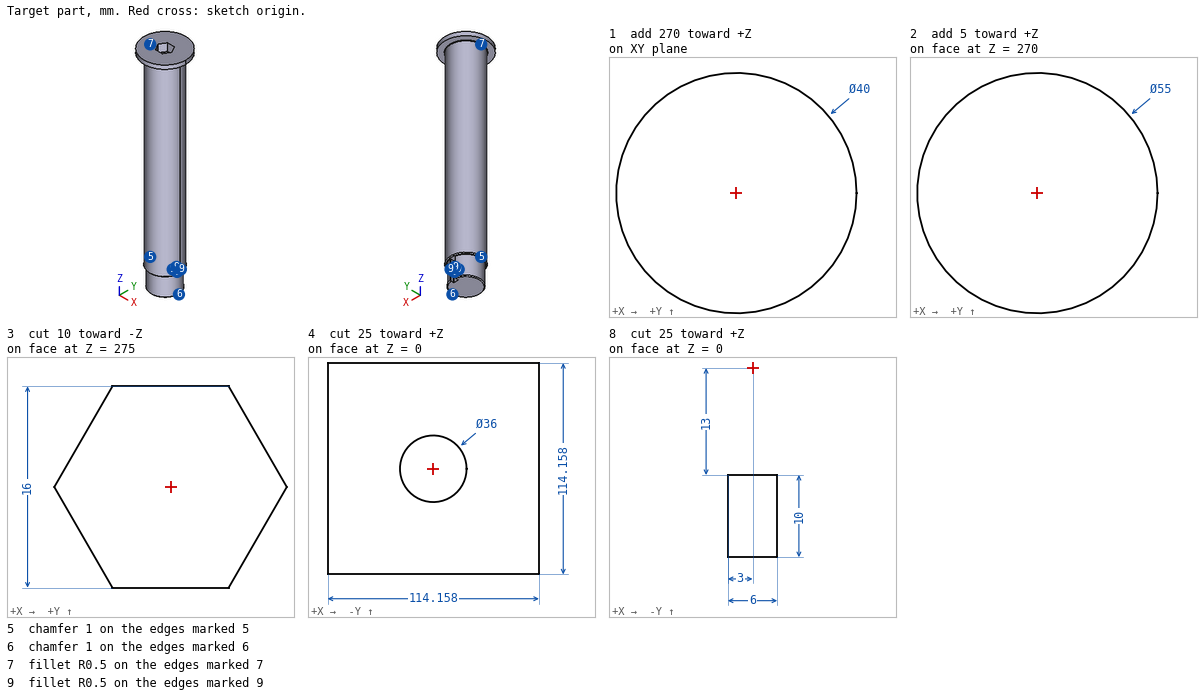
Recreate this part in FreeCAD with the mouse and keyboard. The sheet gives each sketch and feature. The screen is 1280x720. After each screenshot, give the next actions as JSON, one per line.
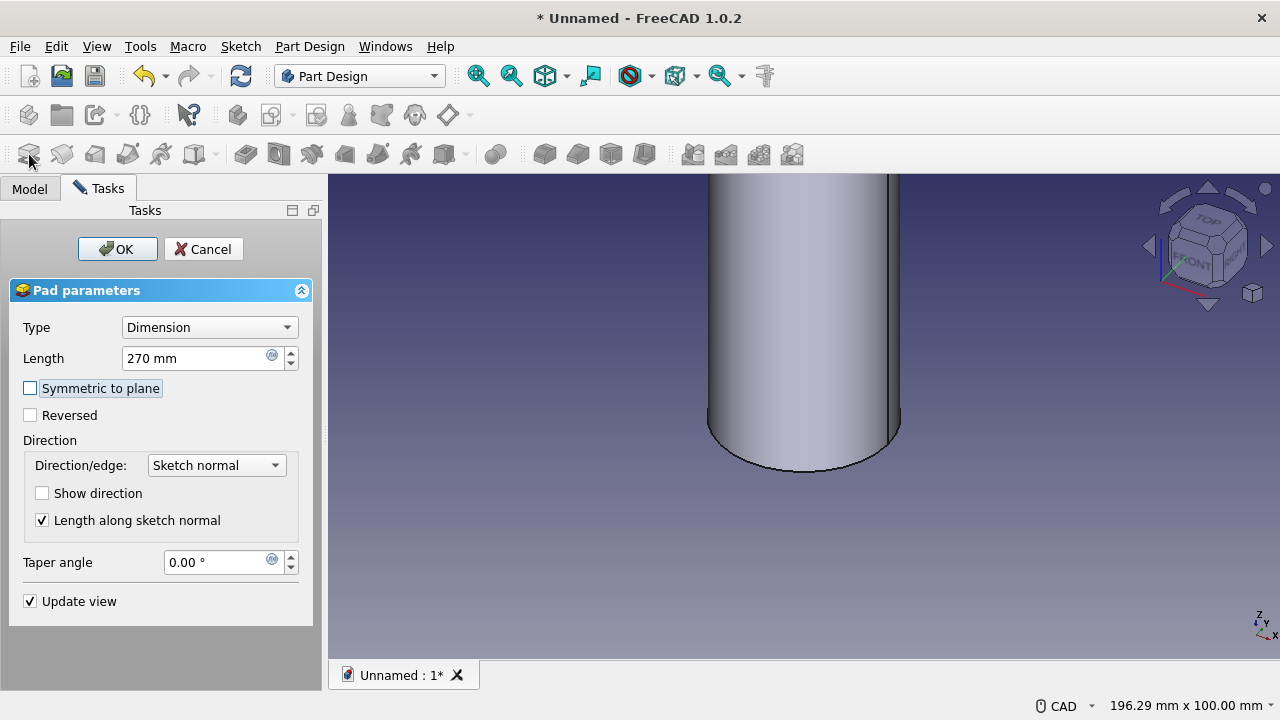
{"action": "left_click", "coordinate": [118, 249]}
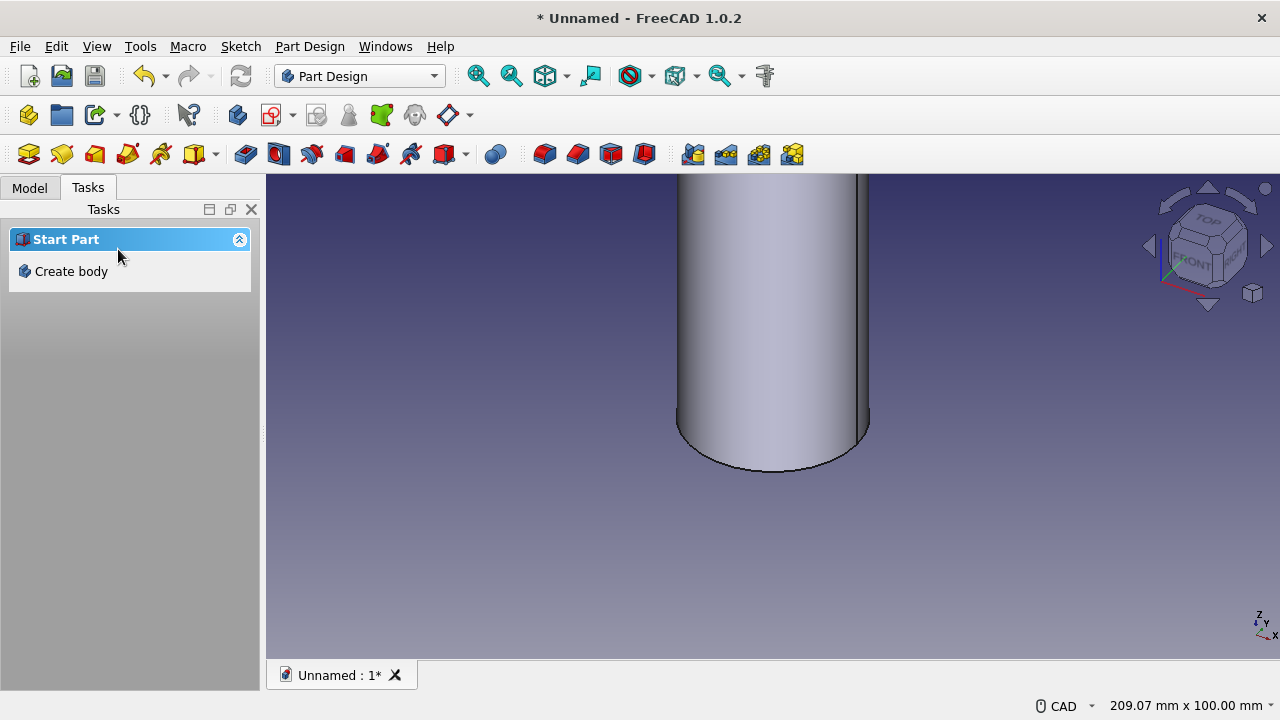
{"action": "left_click", "coordinate": [479, 76]}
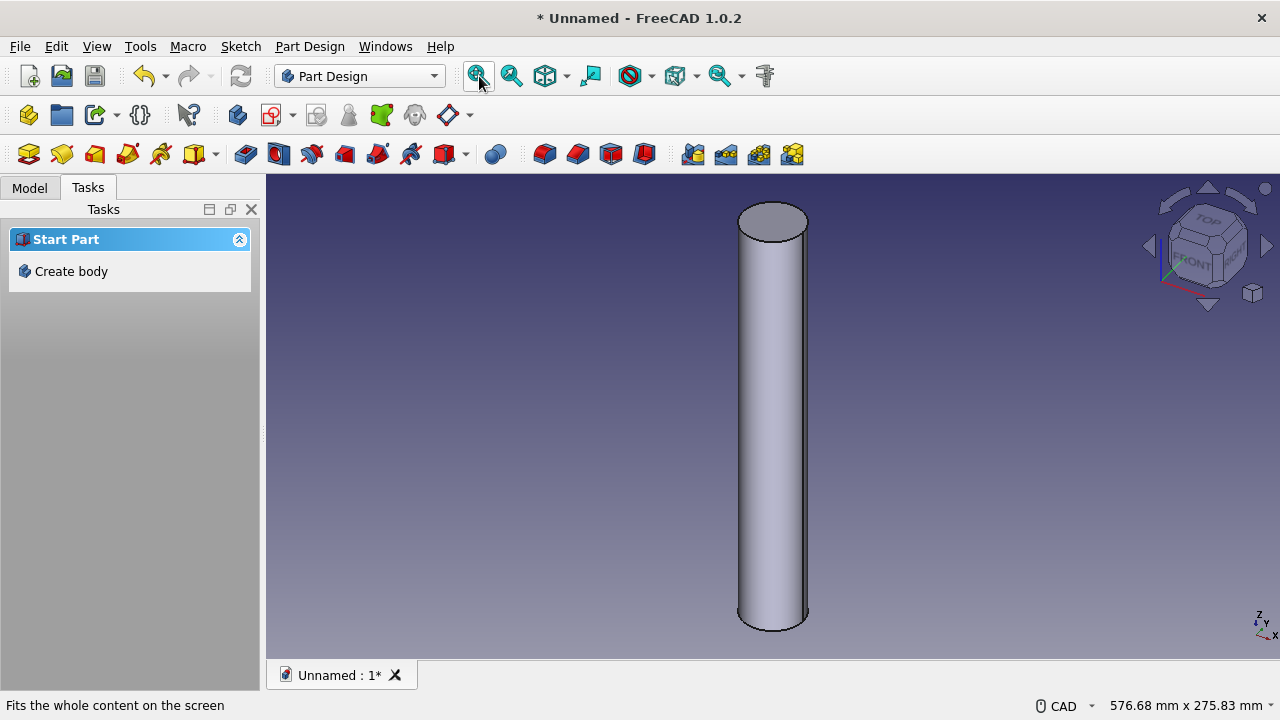
{"action": "left_click", "coordinate": [773, 221]}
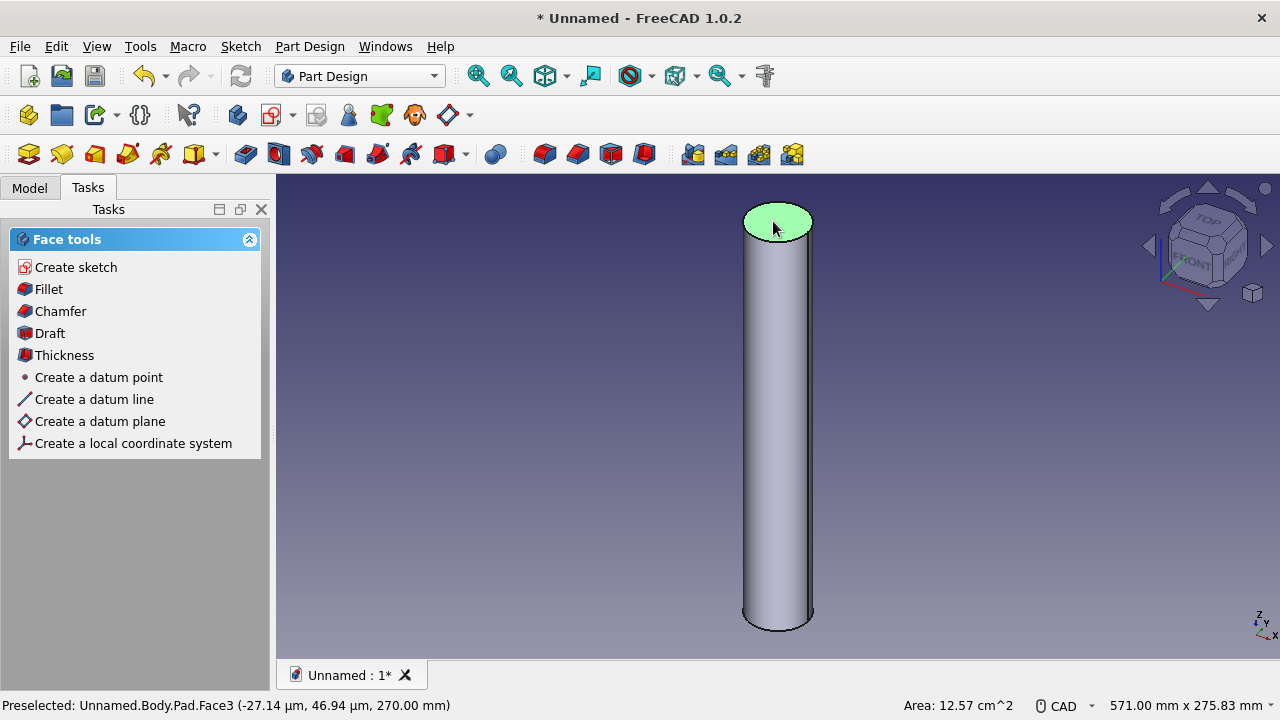
{"action": "left_click", "coordinate": [270, 116]}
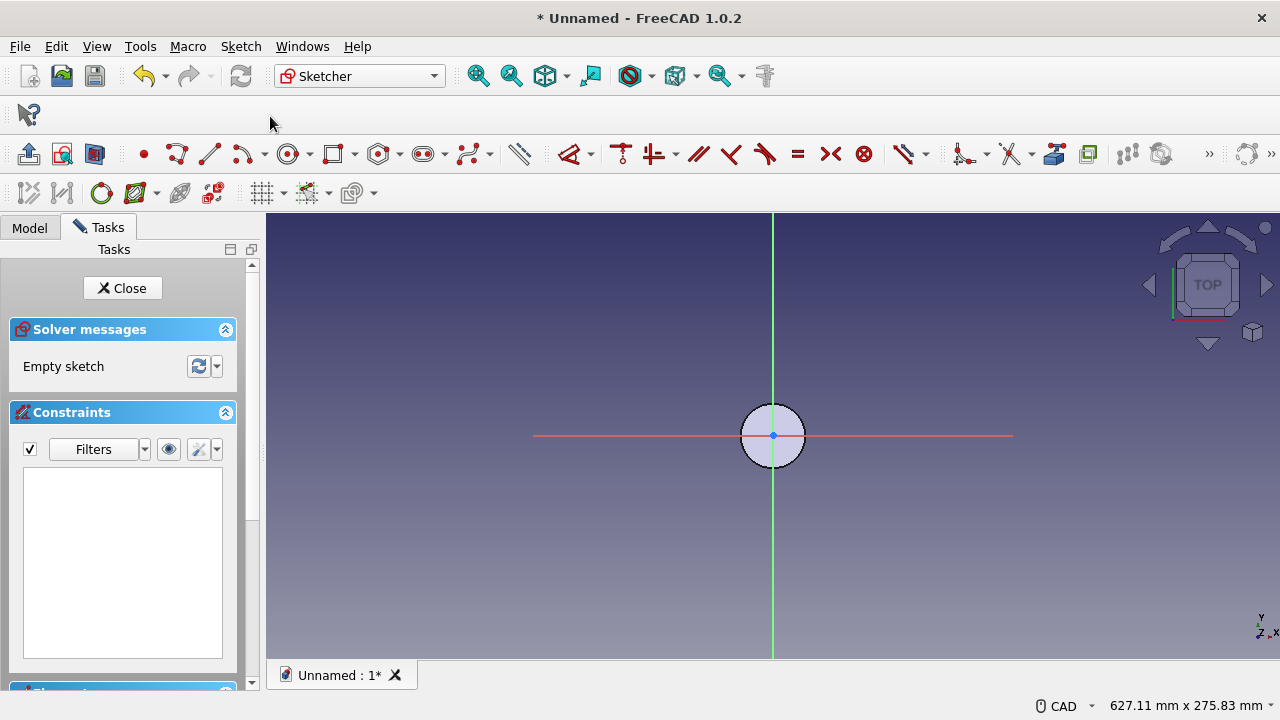
{"action": "scroll", "coordinate": [803, 436], "scroll_direction": "up", "scroll_amount": 6}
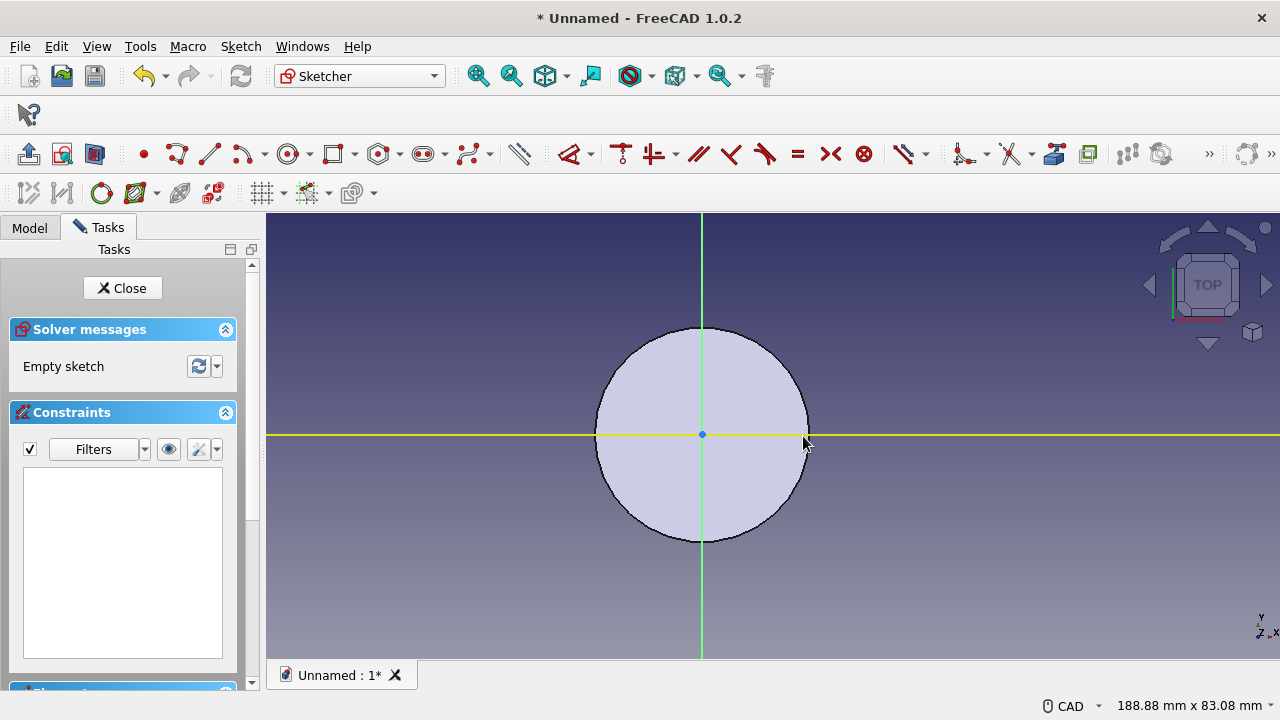
{"action": "left_click", "coordinate": [288, 154]}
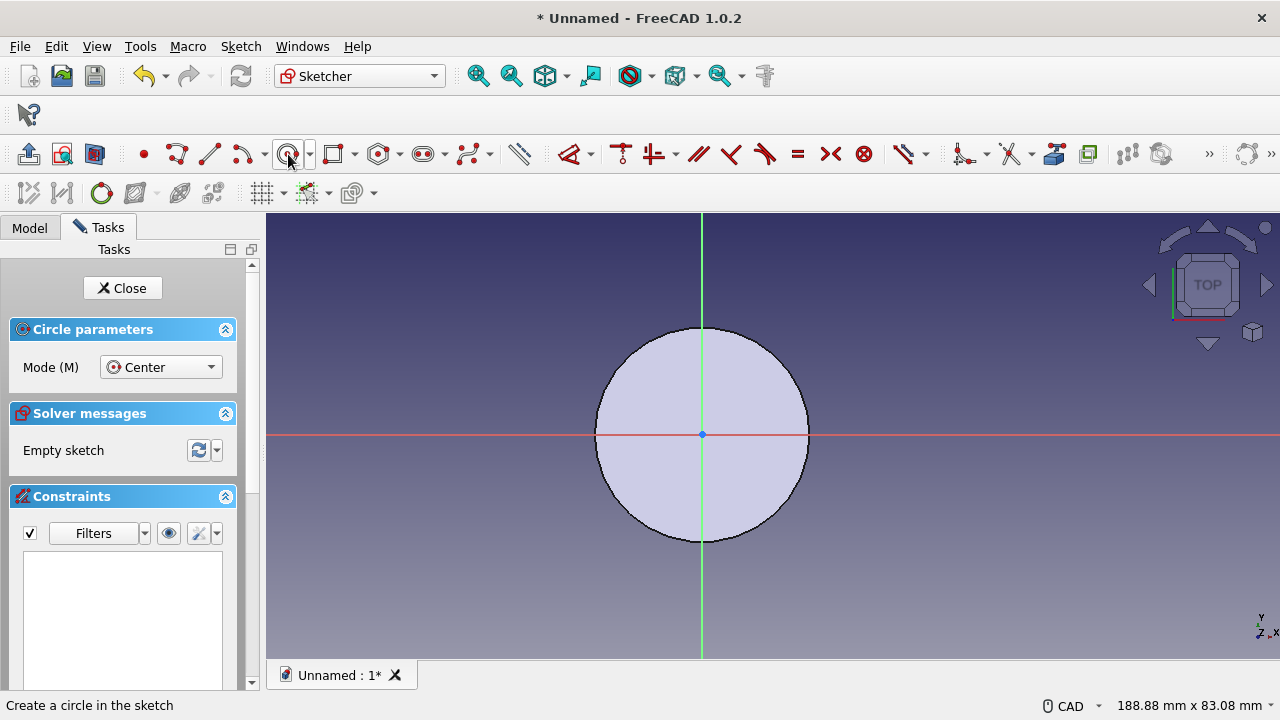
{"action": "left_click", "coordinate": [702, 435]}
{"action": "mouse_move", "coordinate": [807, 330]}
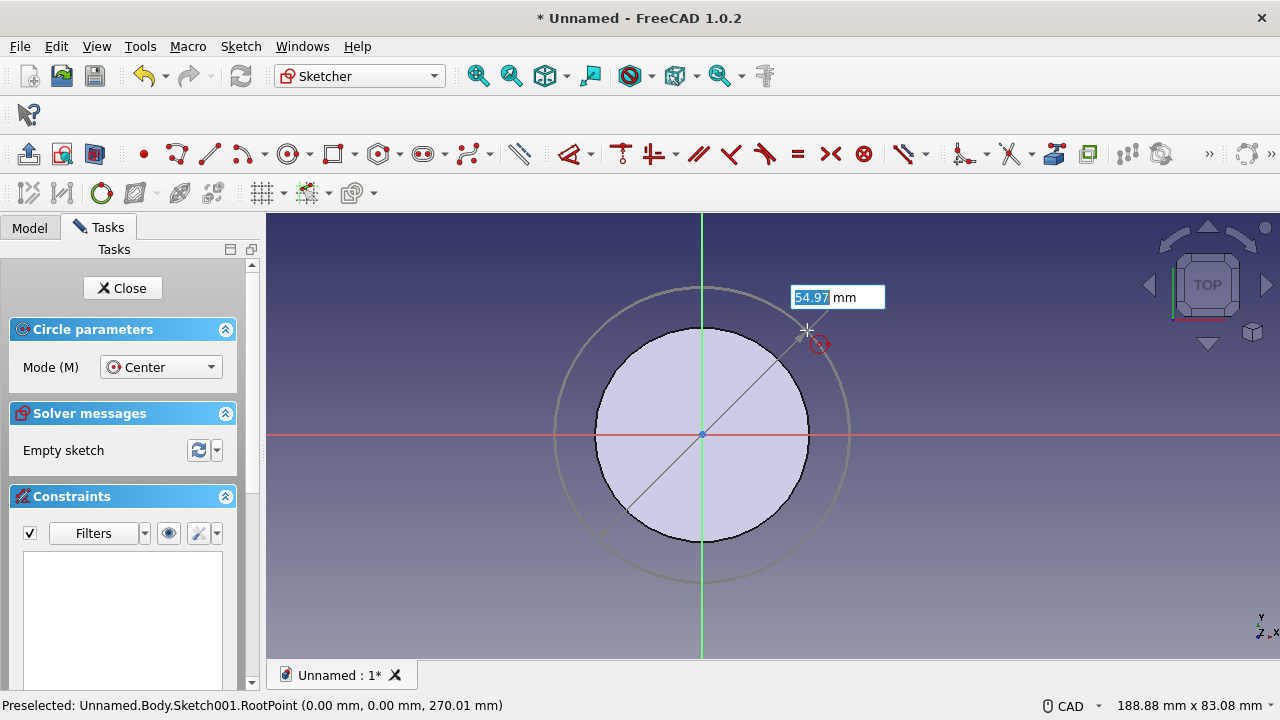
{"action": "type", "text": "55"}
{"action": "key", "text": "Return"}
{"action": "key", "text": "Escape"}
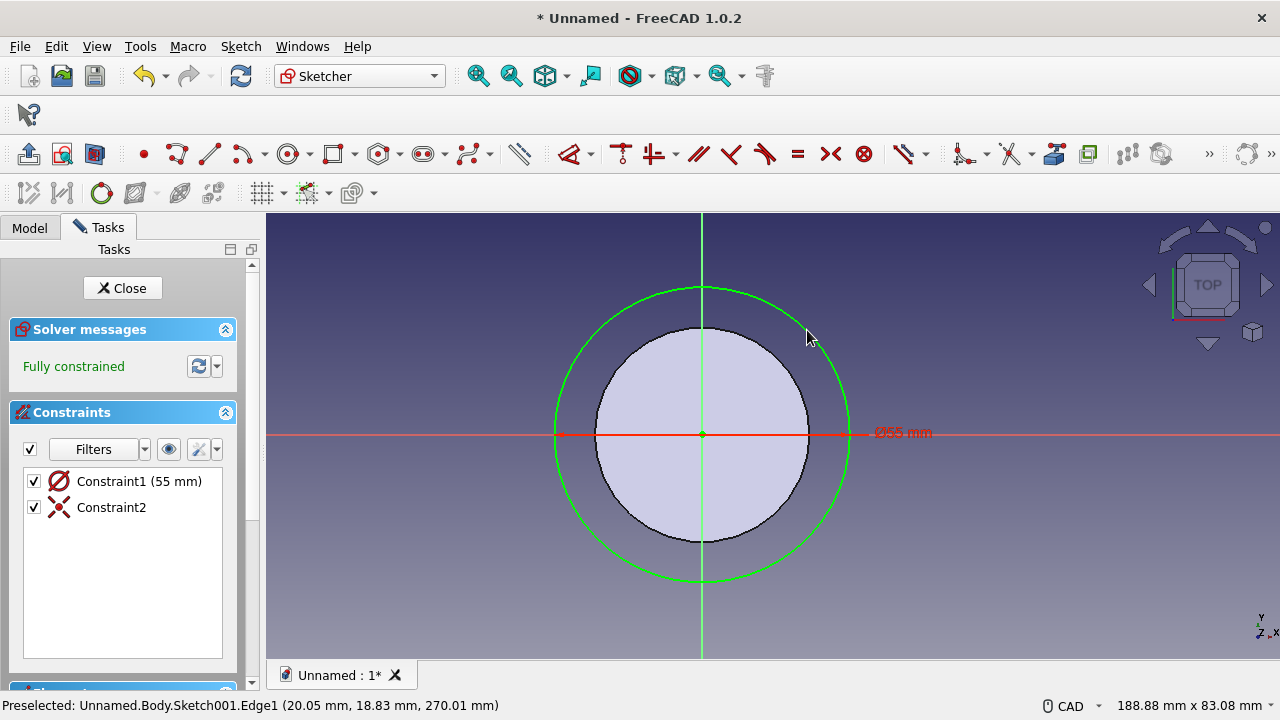
{"action": "left_click", "coordinate": [123, 288]}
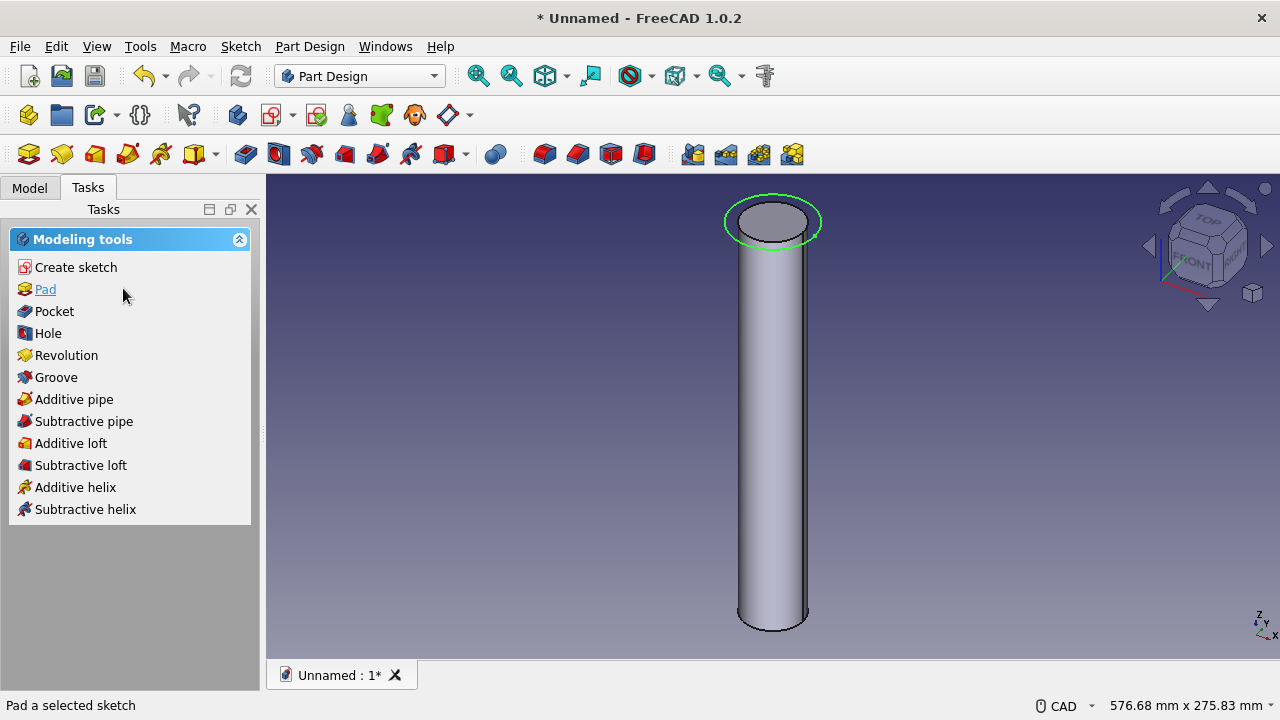
{"action": "left_click", "coordinate": [29, 154]}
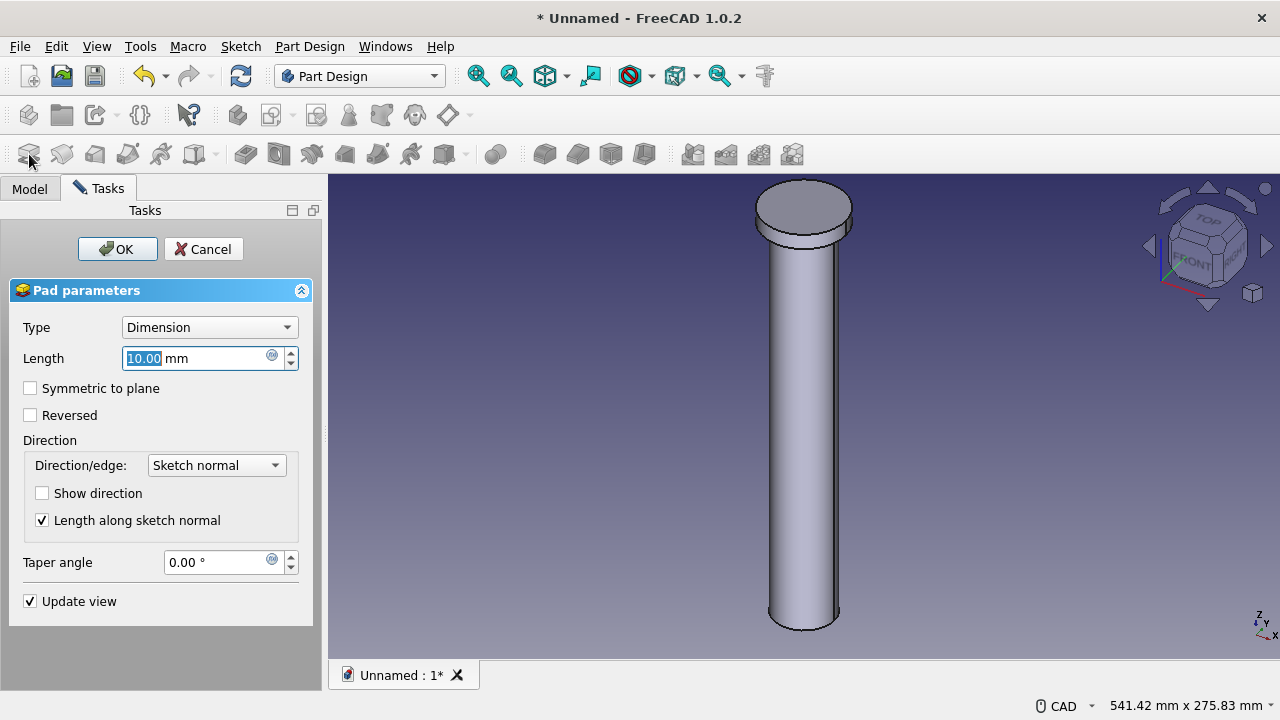
{"action": "type", "text": "5"}
{"action": "key", "text": "Tab"}